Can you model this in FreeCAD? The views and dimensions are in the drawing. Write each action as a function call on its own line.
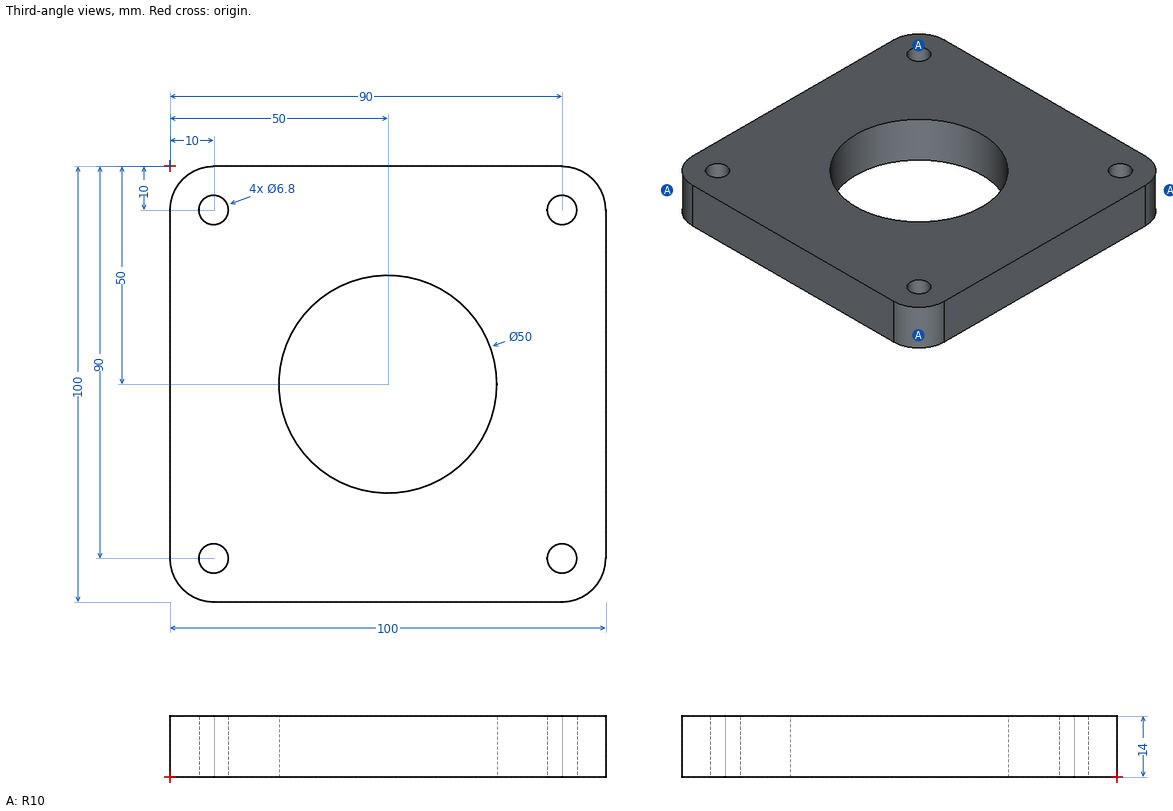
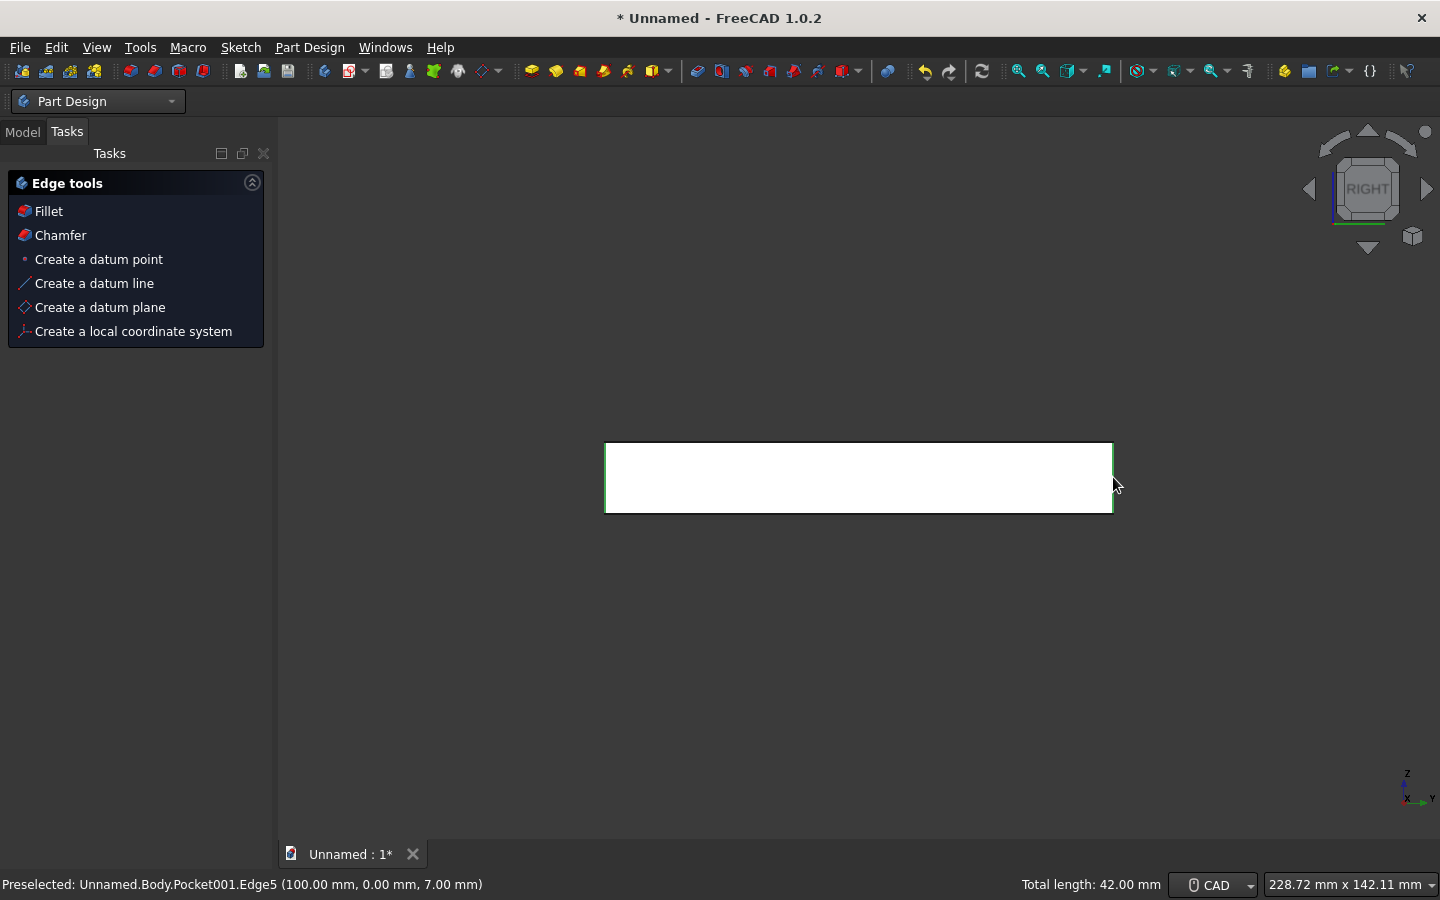
key(5)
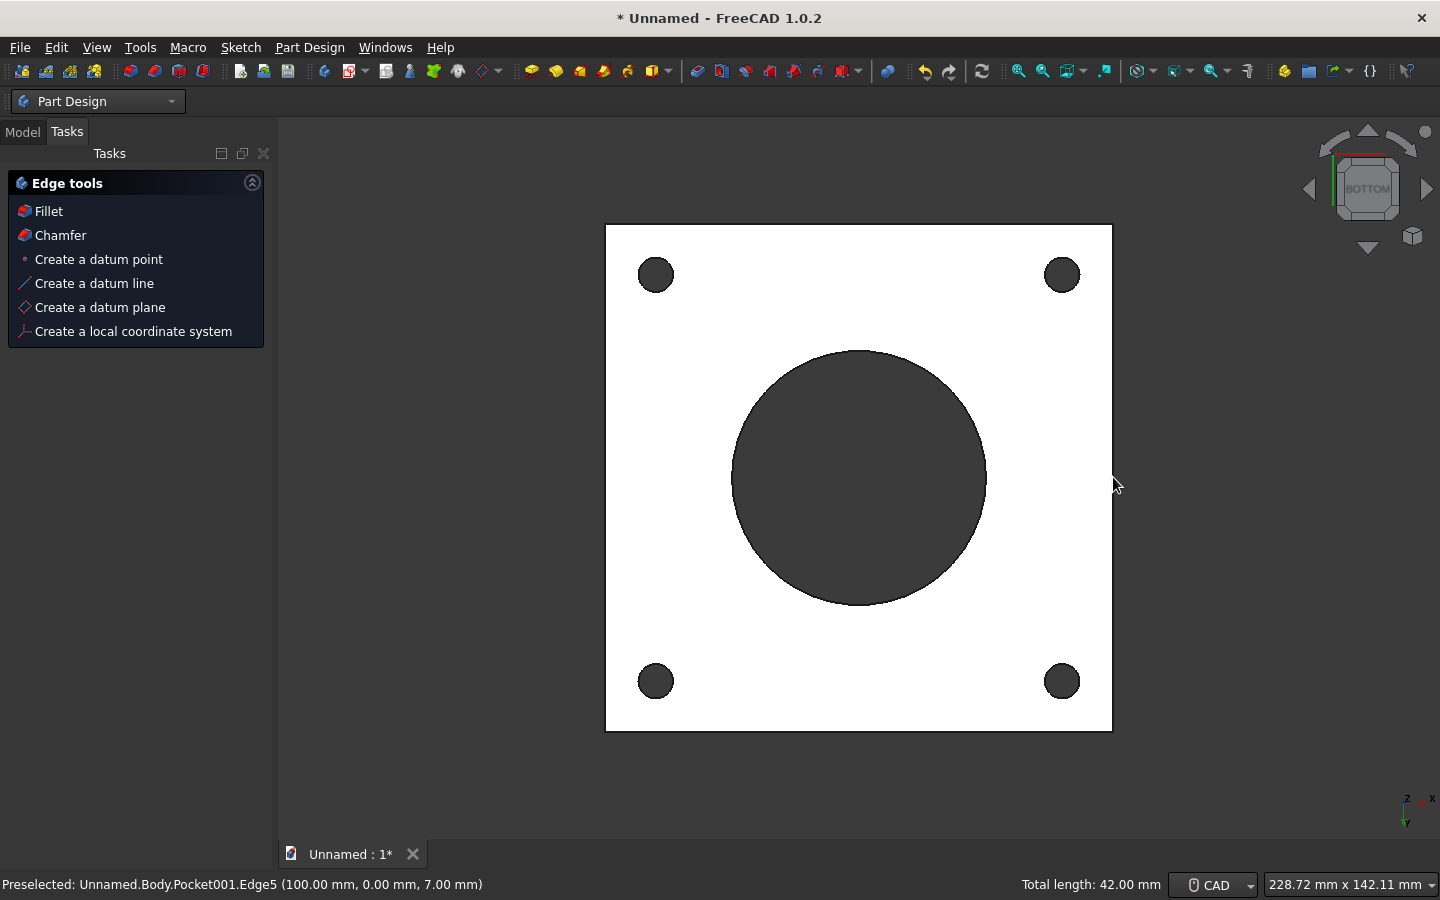
key(4)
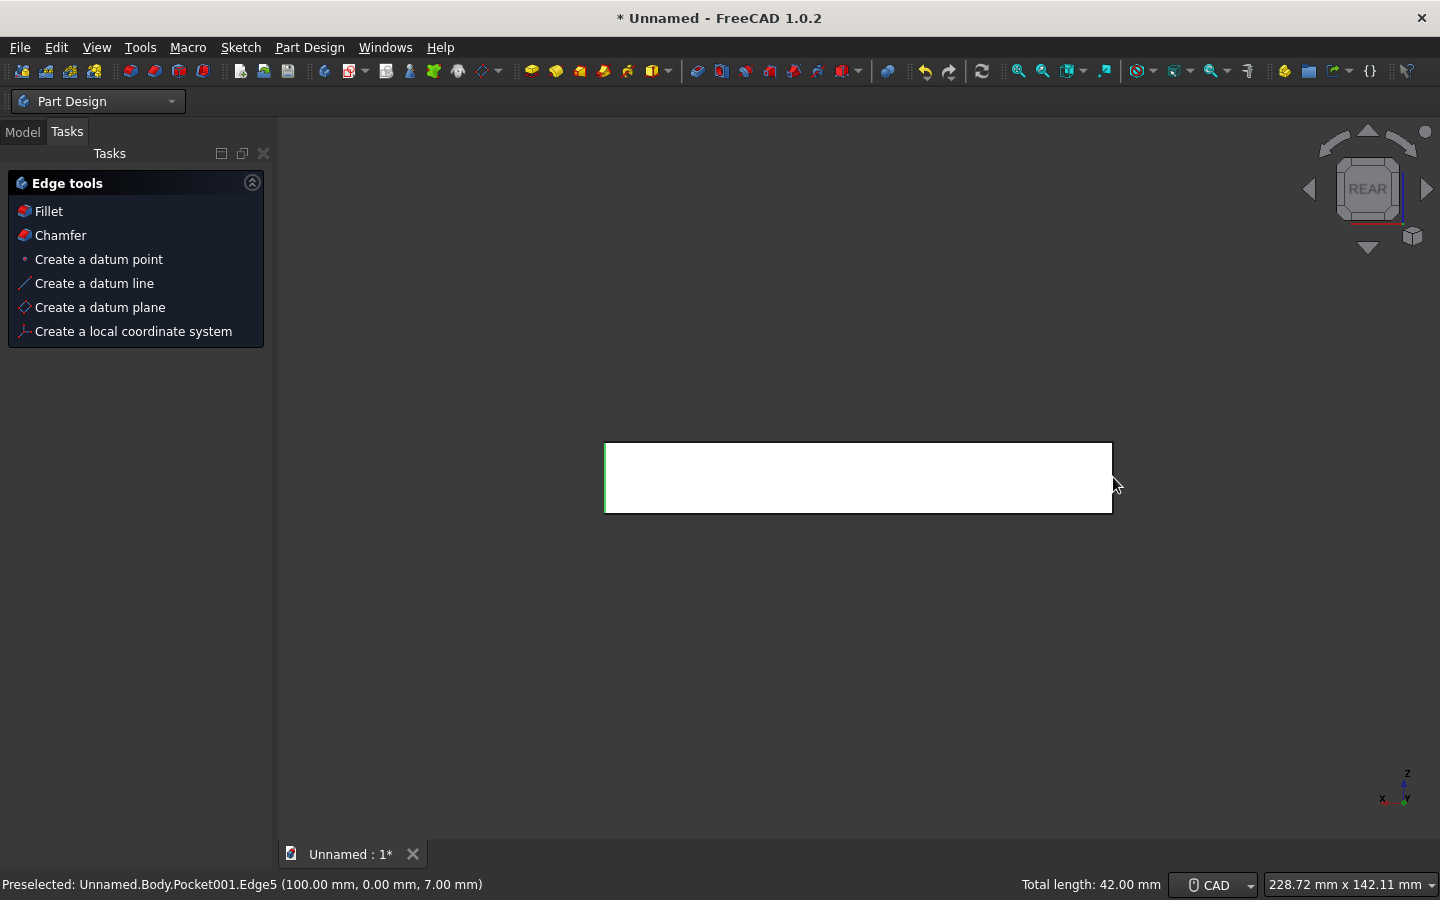
click(1020, 72)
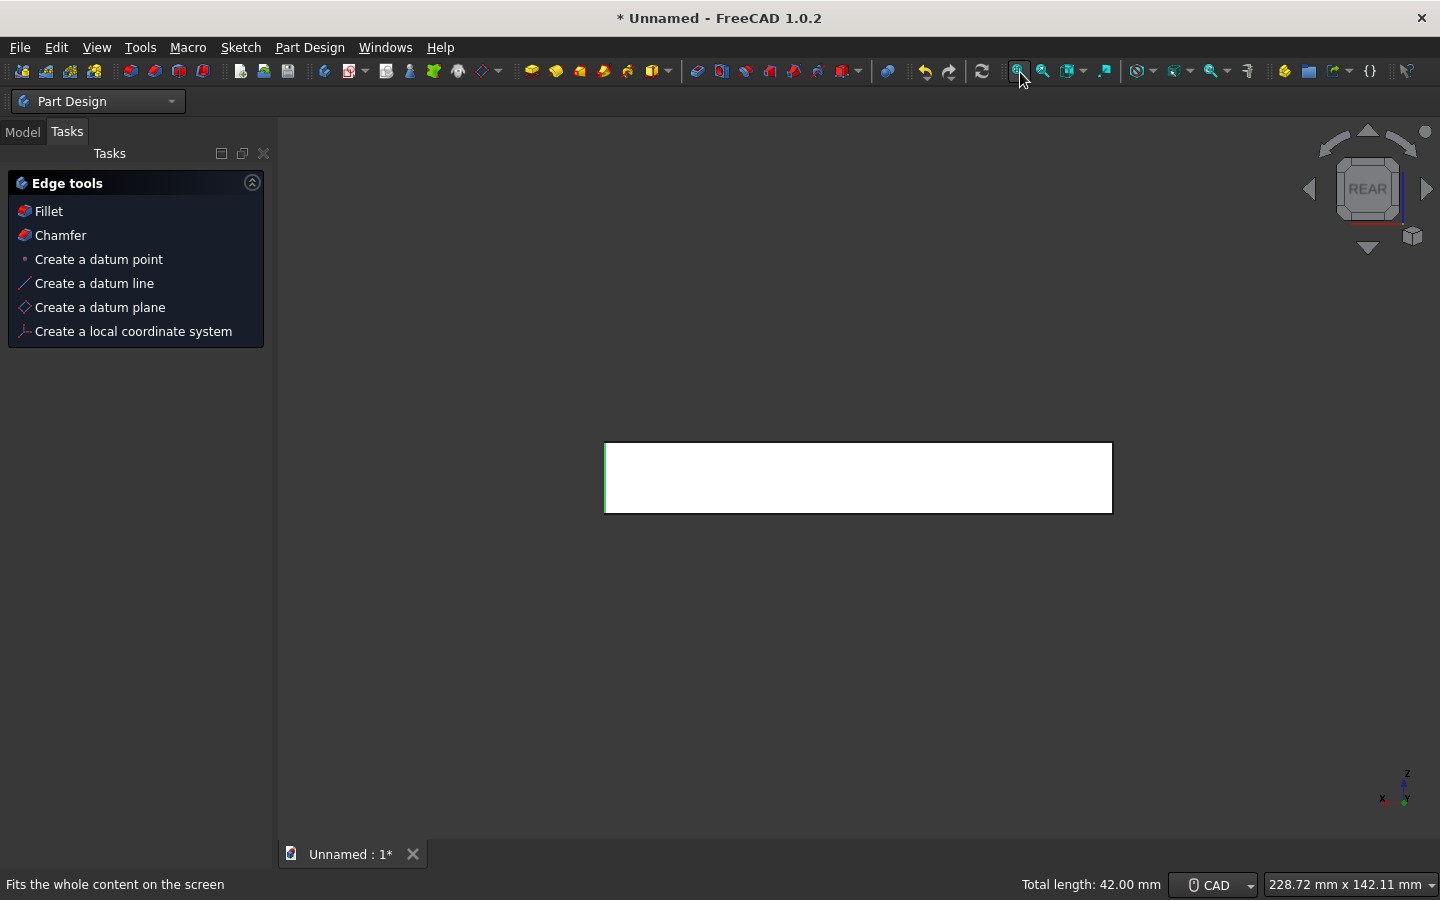
click(1113, 477, ctrl)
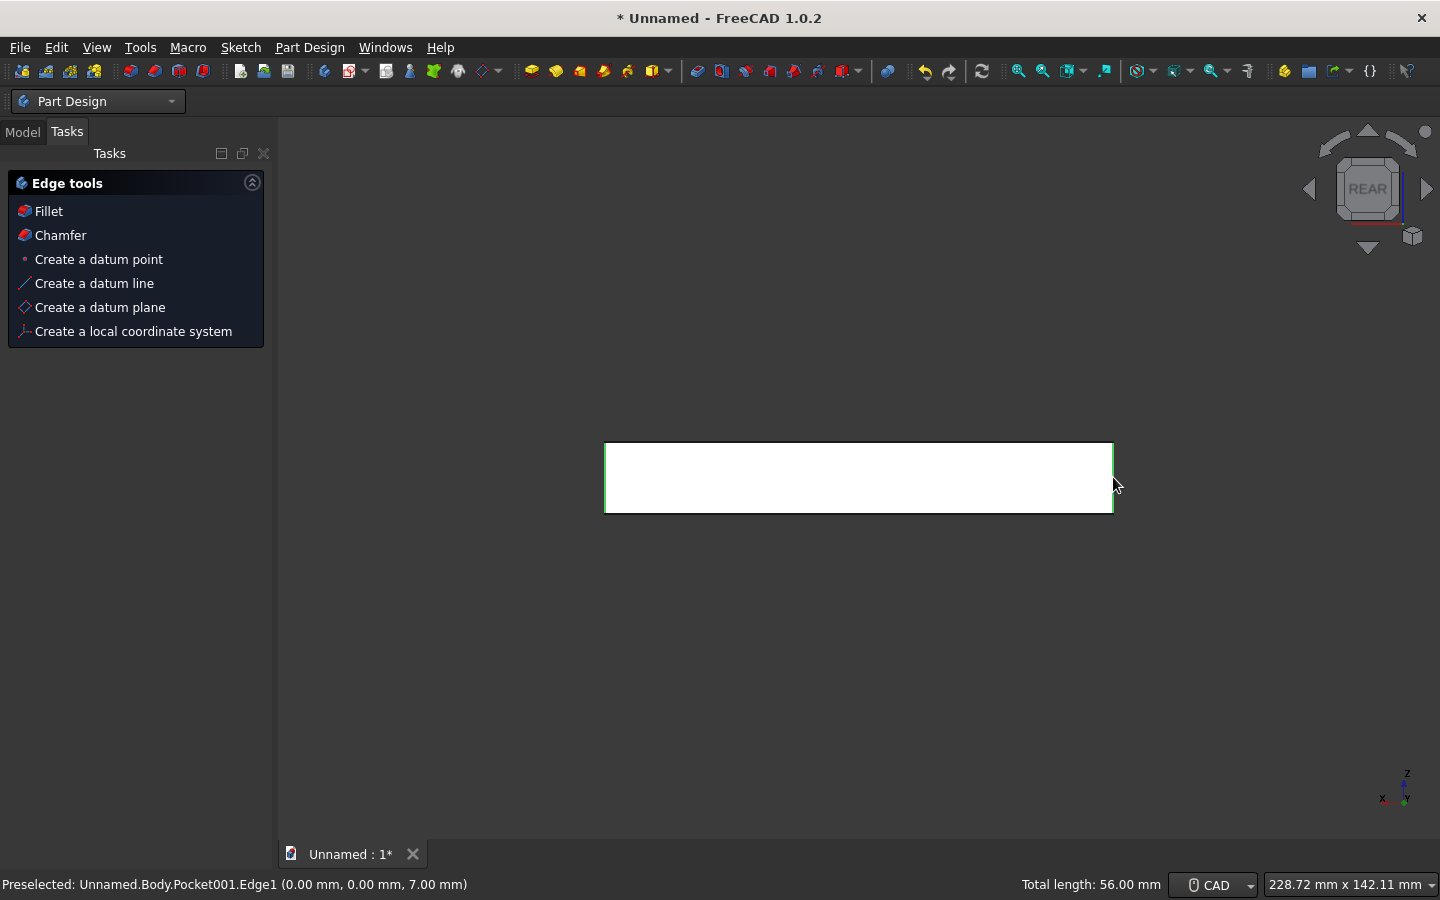
click(132, 72)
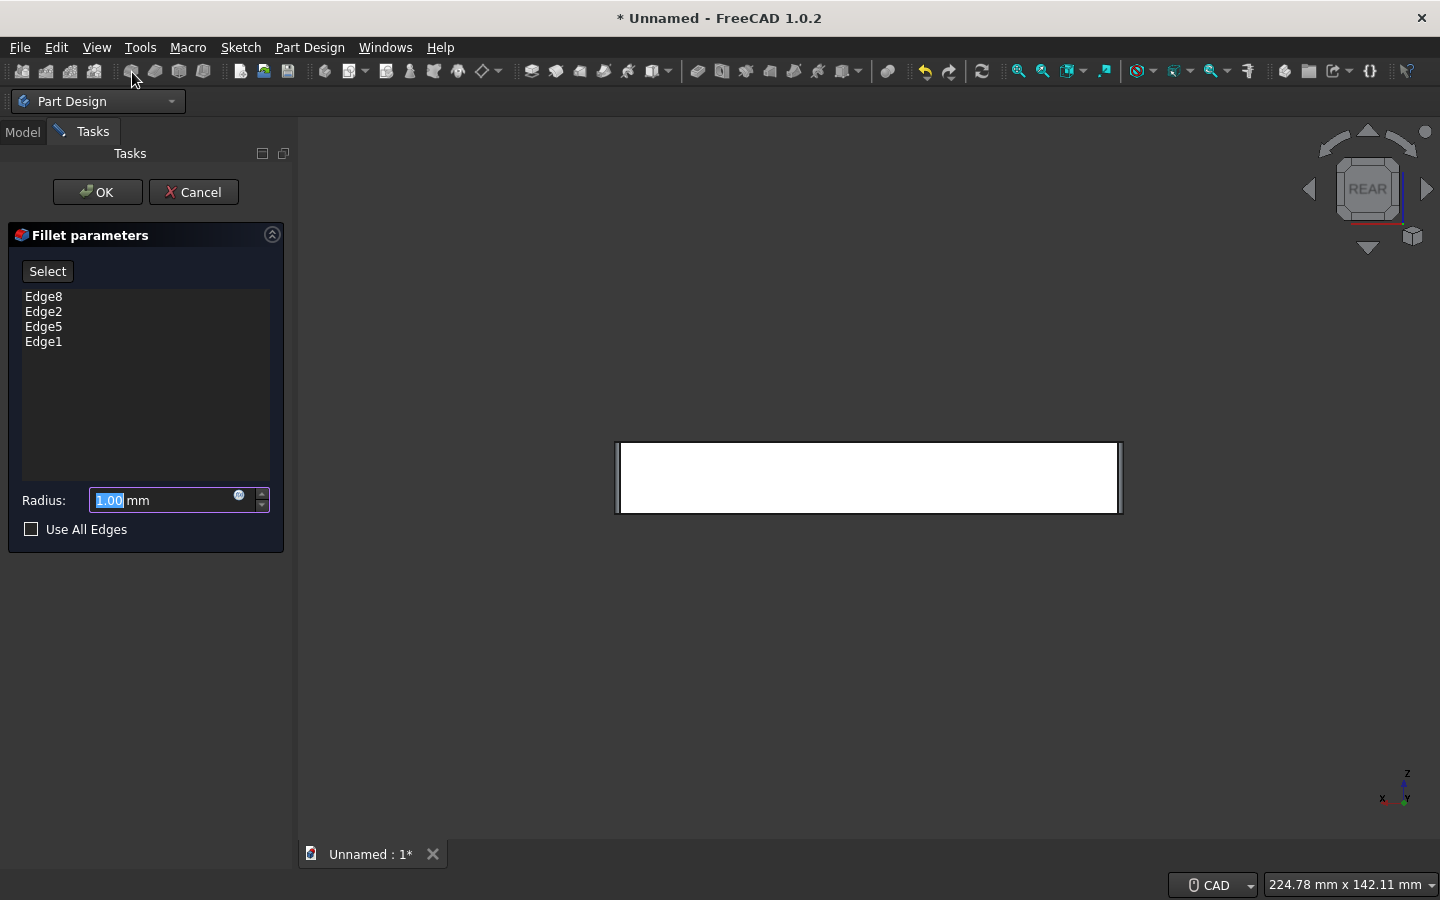
text(10)
key(Tab)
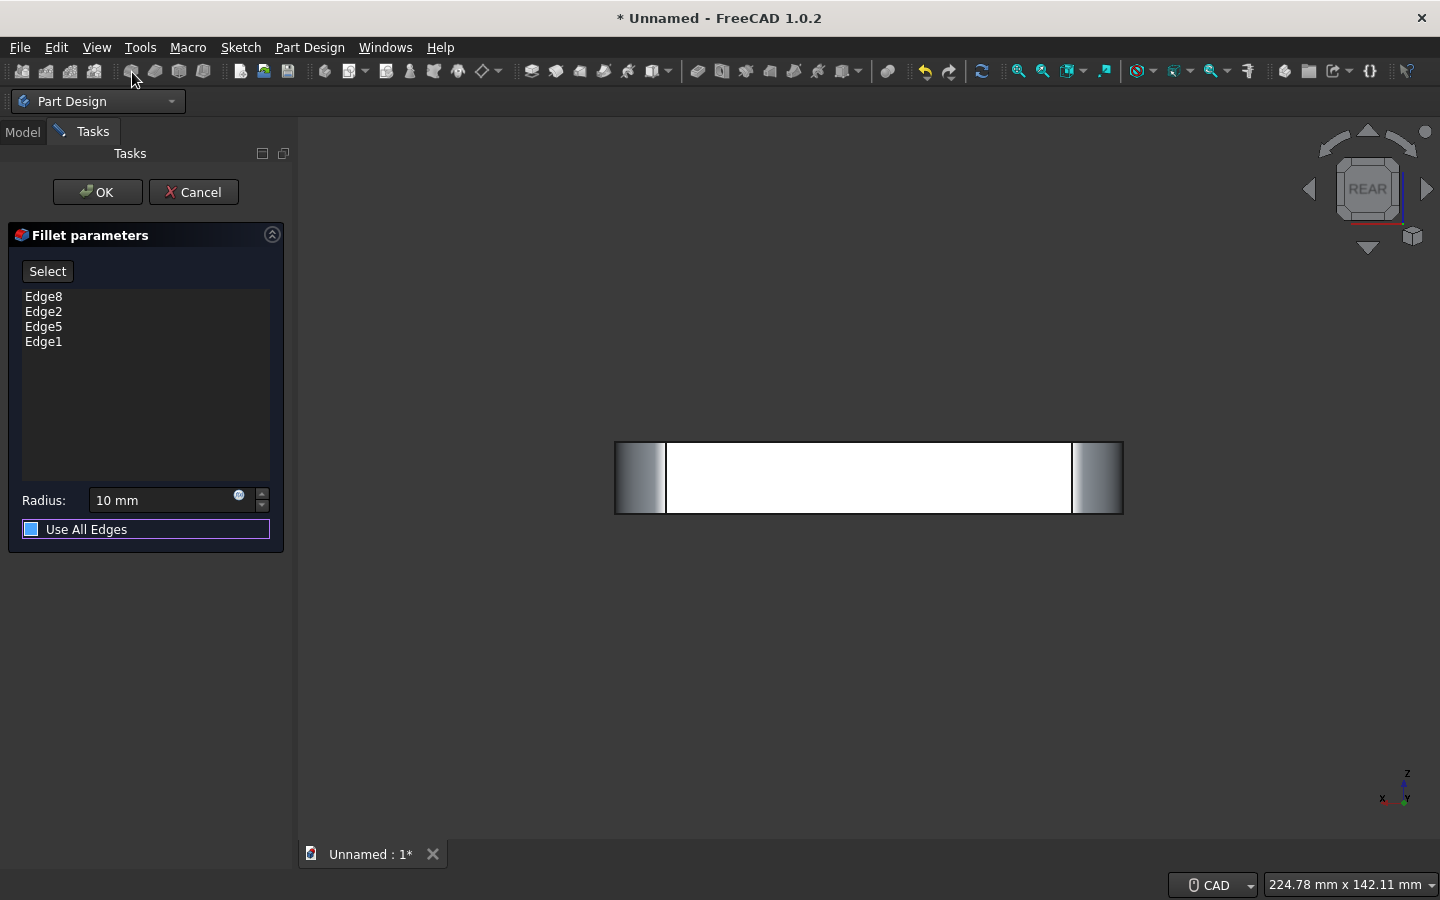
click(98, 192)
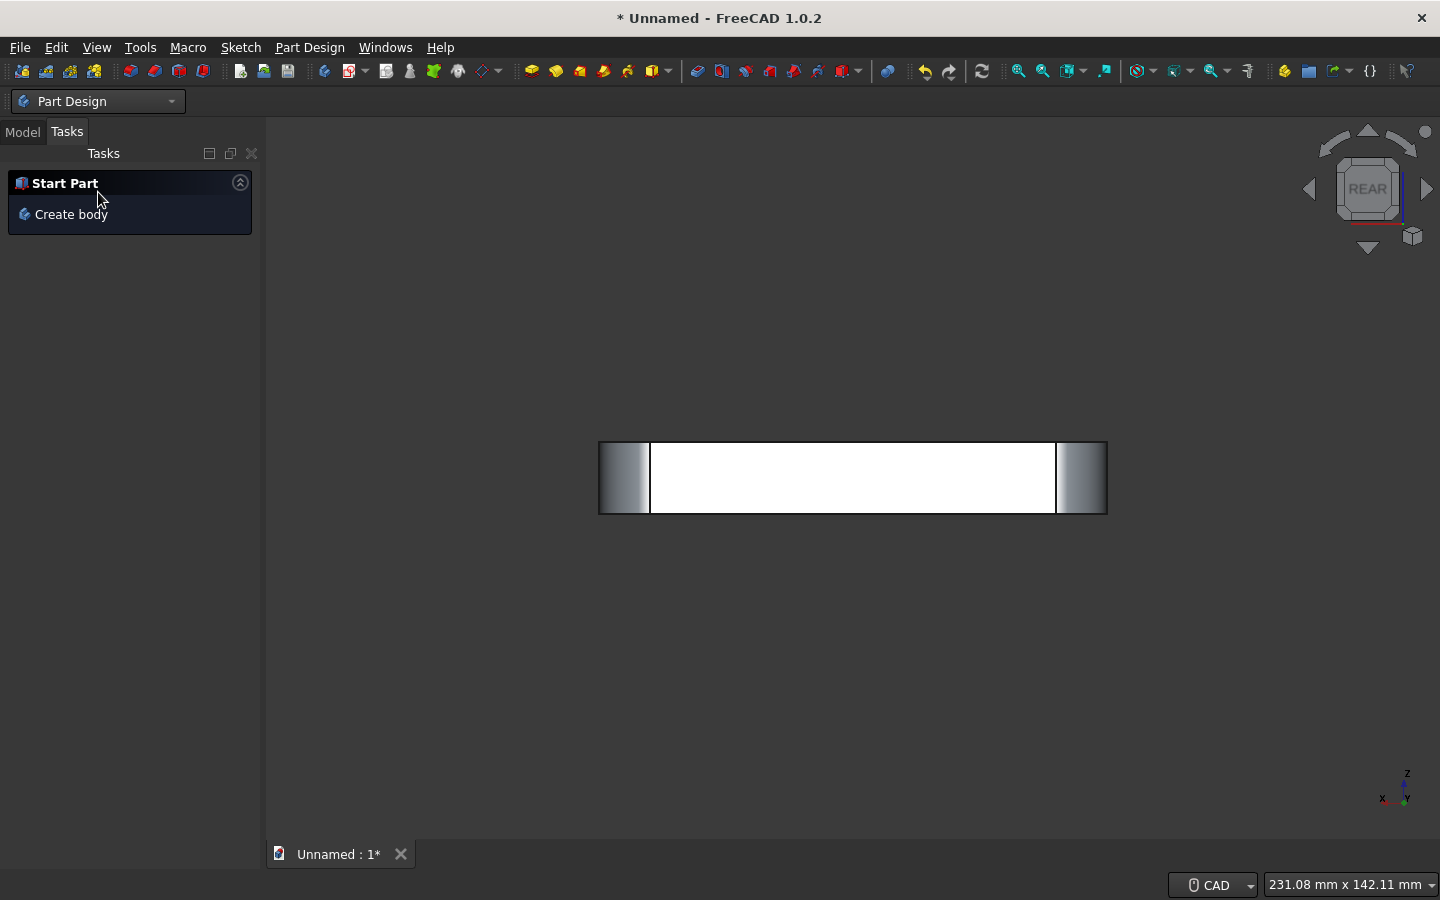
key(0)